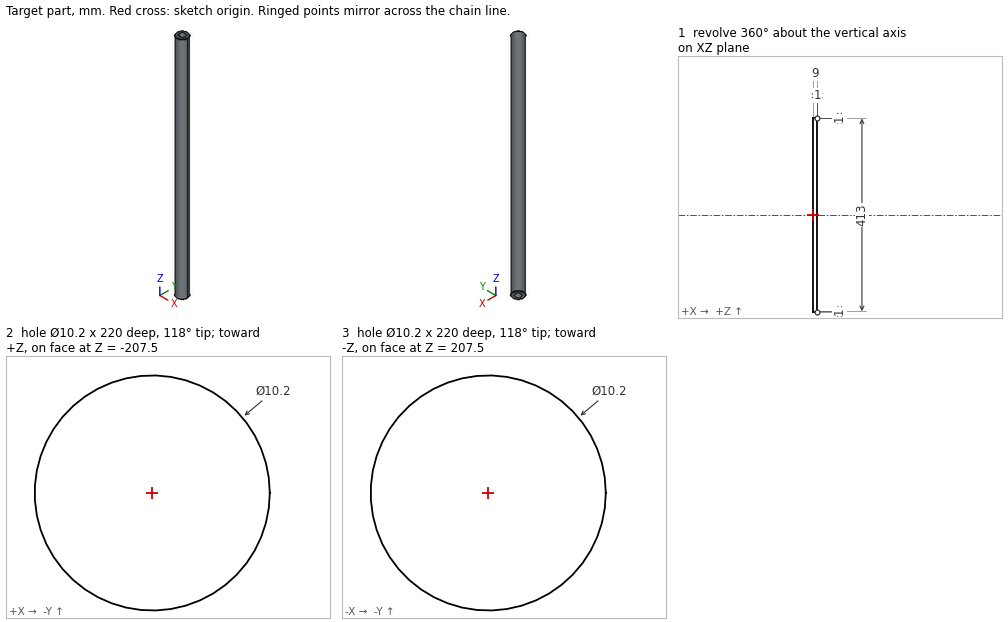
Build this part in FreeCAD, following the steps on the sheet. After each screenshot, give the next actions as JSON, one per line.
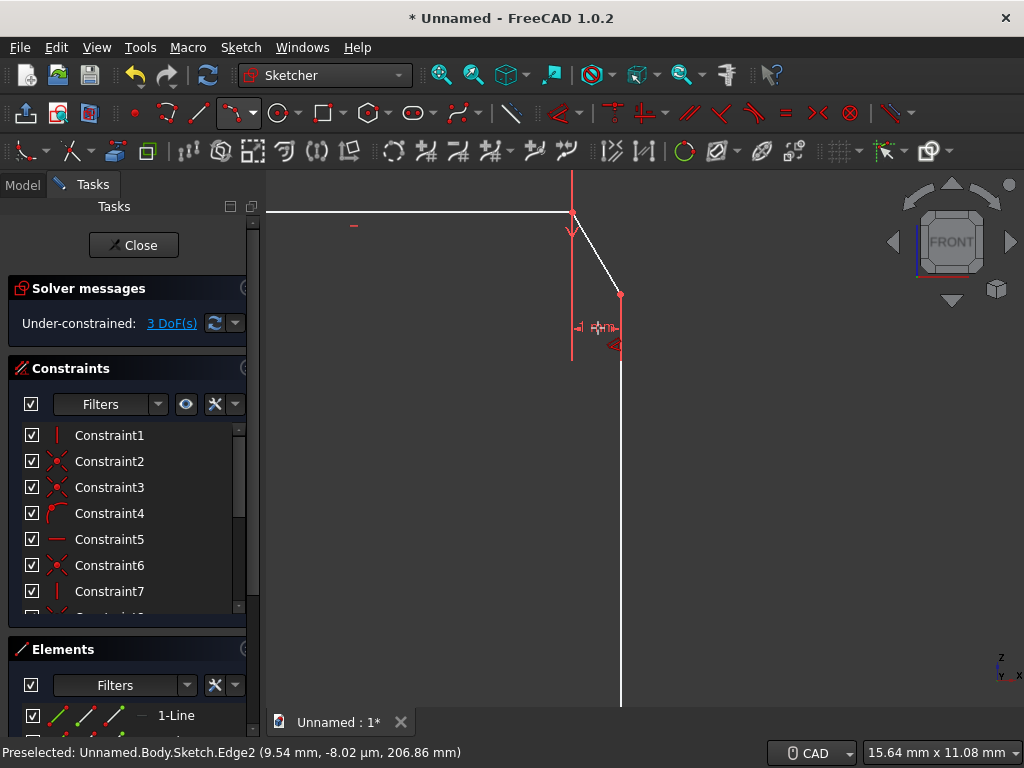
{"action": "left_click", "coordinate": [606, 270]}
{"action": "left_click", "coordinate": [655, 253]}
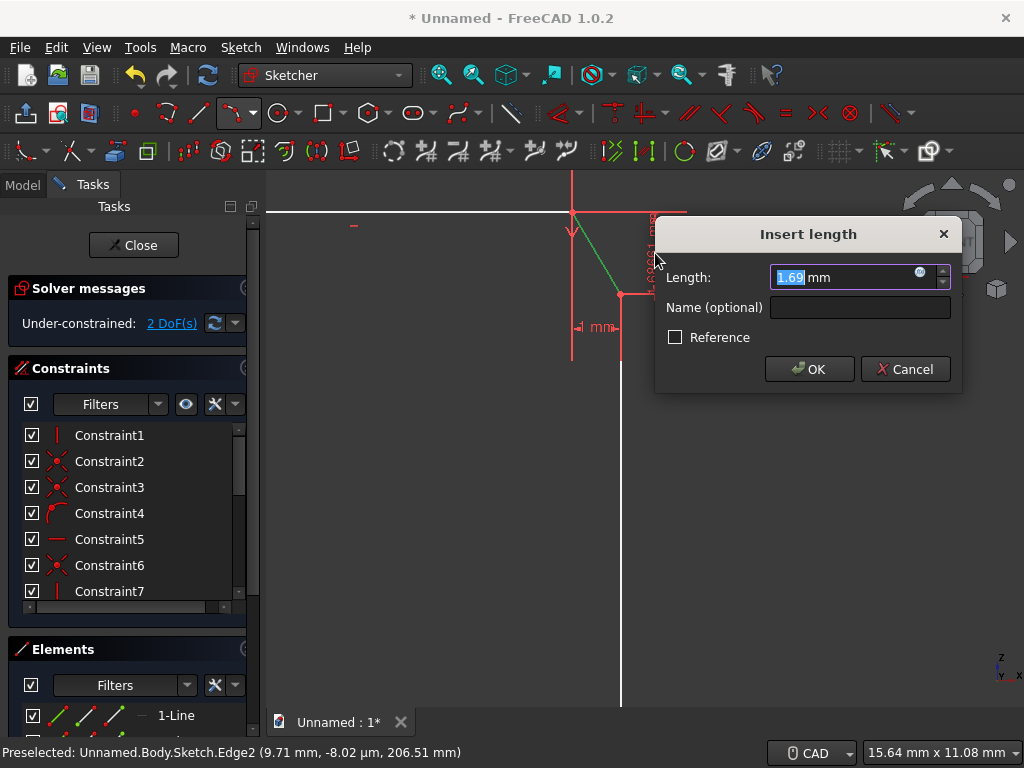
{"action": "type", "text": "1"}
{"action": "key", "text": "Return"}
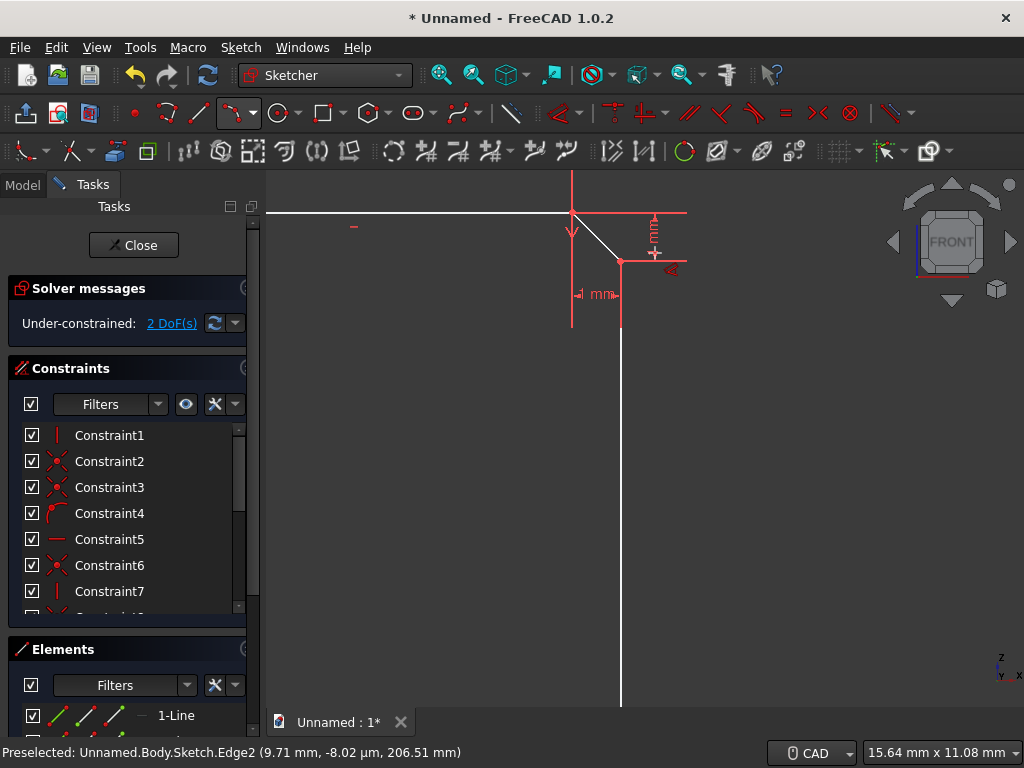
{"action": "scroll", "coordinate": [576, 438], "scroll_direction": "down", "scroll_amount": 15}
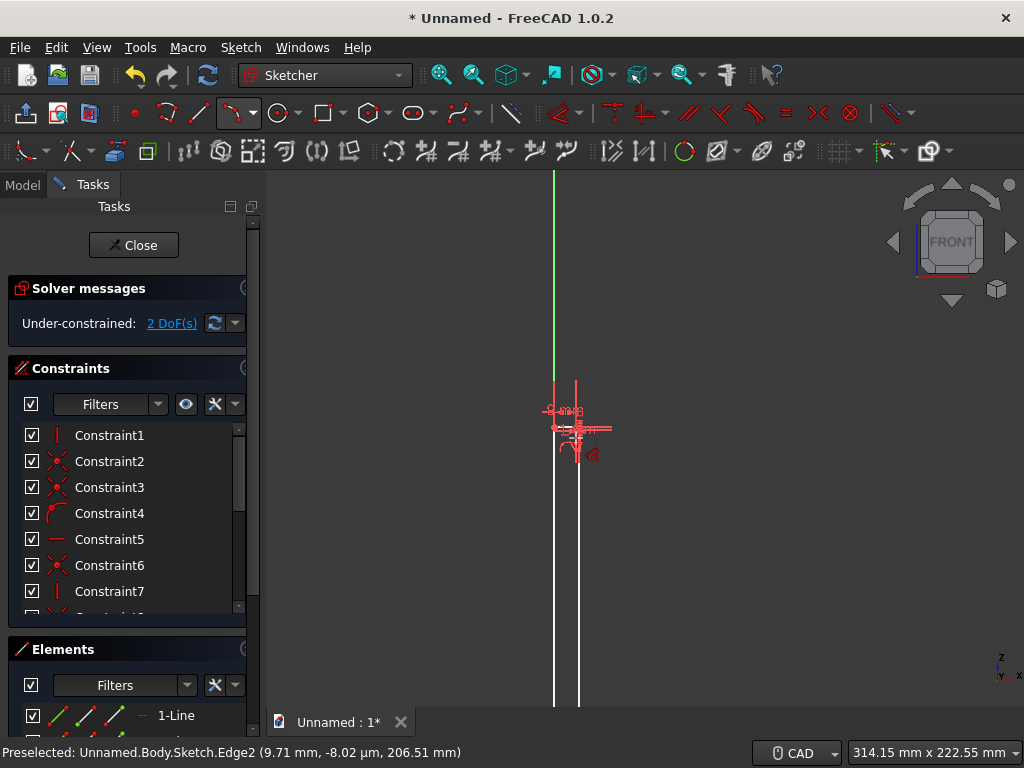
{"action": "scroll", "coordinate": [582, 198], "scroll_direction": "down", "scroll_amount": 5}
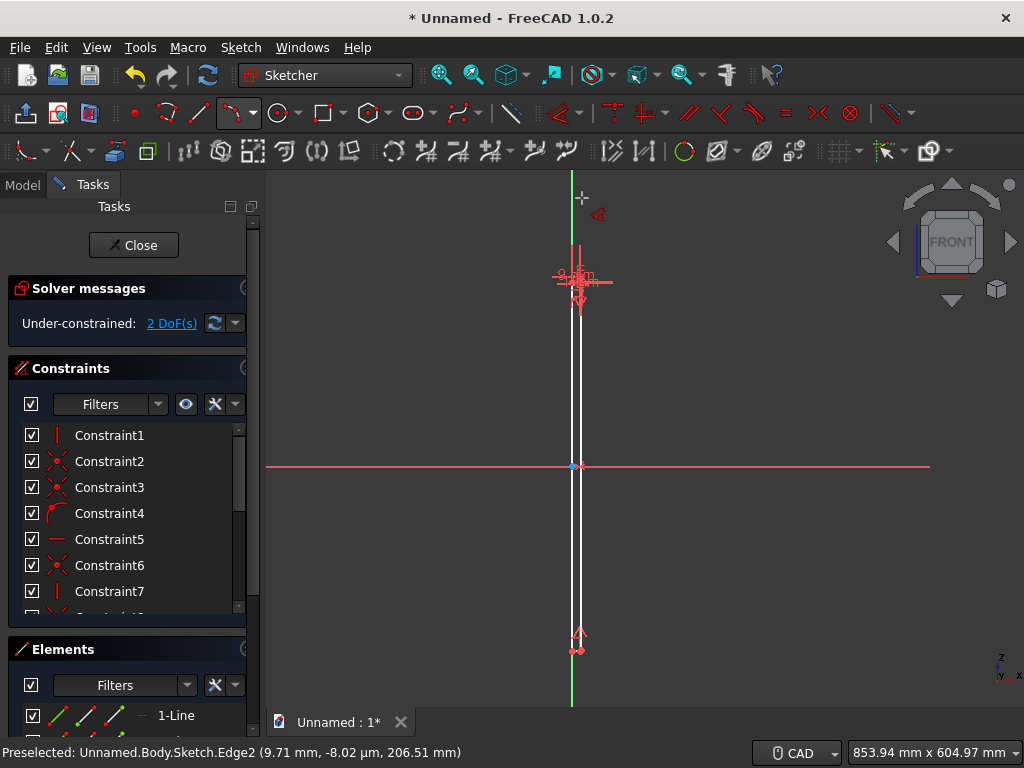
{"action": "scroll", "coordinate": [580, 651], "scroll_direction": "up", "scroll_amount": 20}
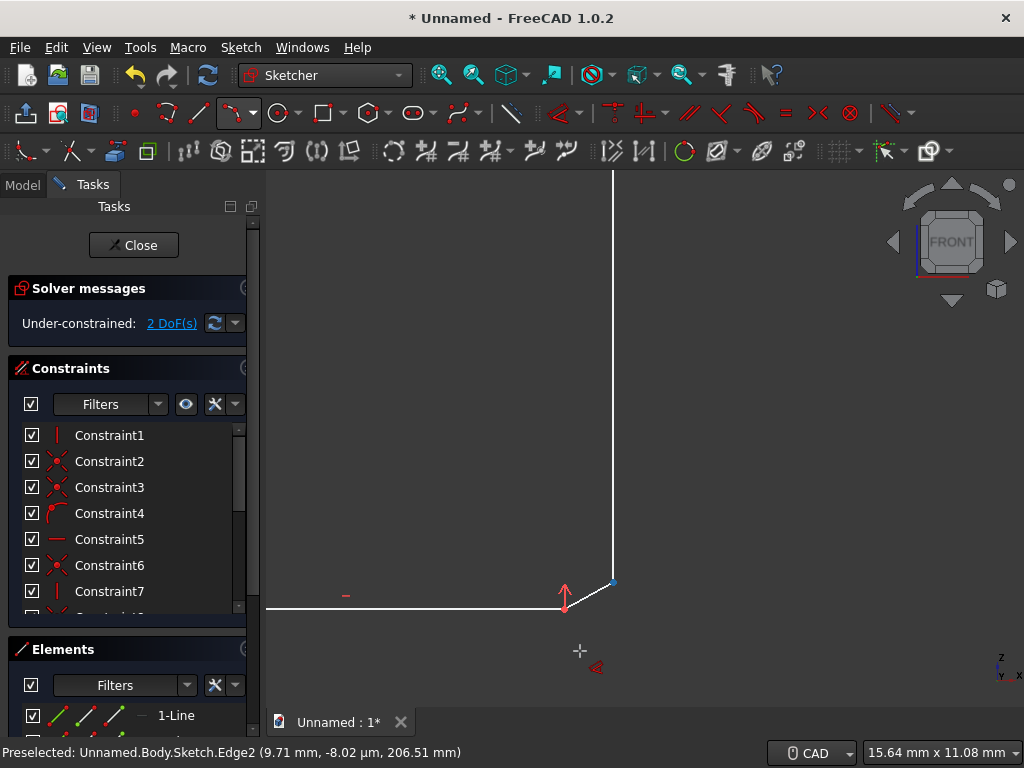
{"action": "left_click", "coordinate": [579, 601]}
{"action": "left_click", "coordinate": [647, 596]}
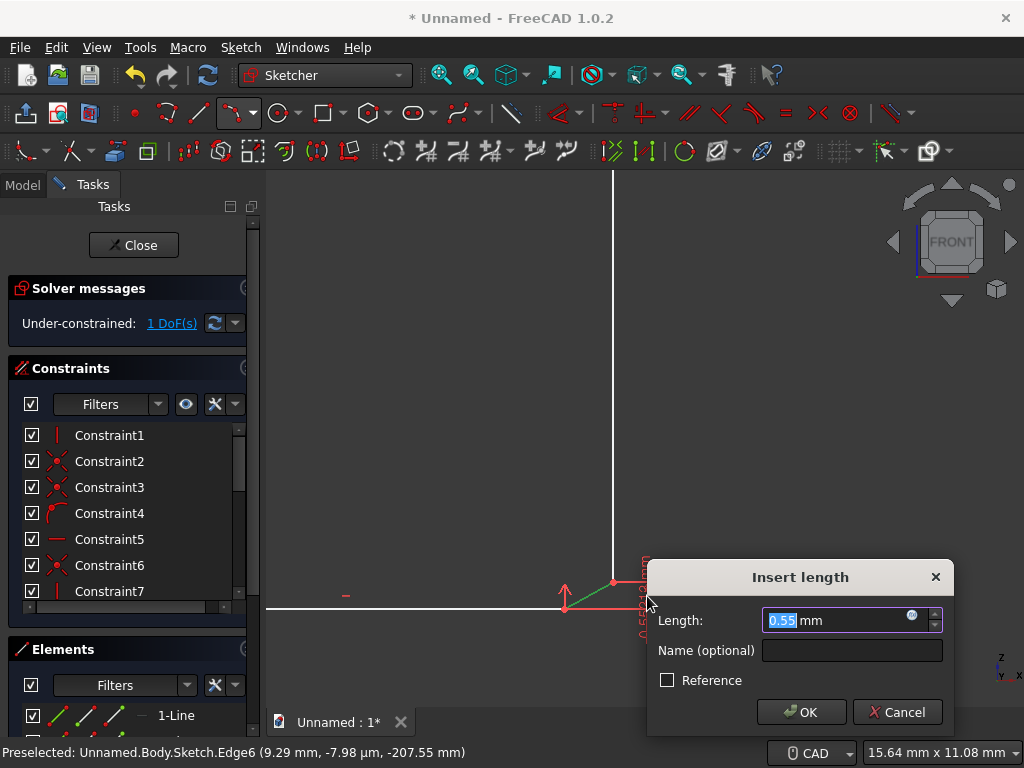
{"action": "type", "text": "1"}
{"action": "key", "text": "Return"}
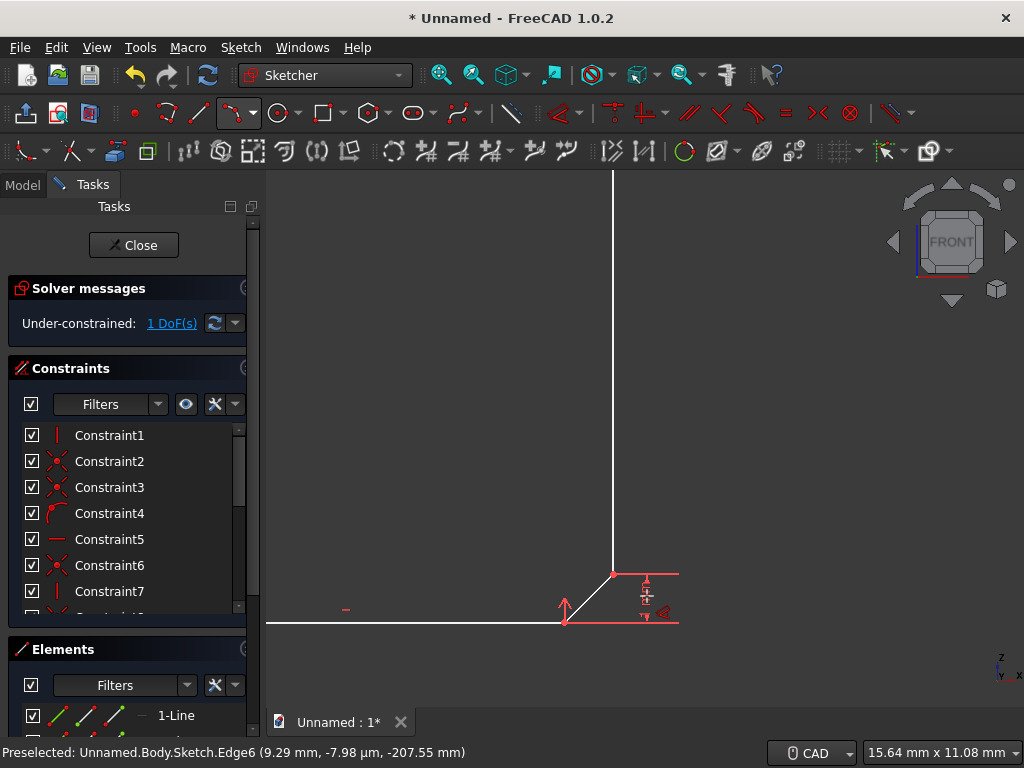
{"action": "scroll", "coordinate": [576, 438], "scroll_direction": "down", "scroll_amount": 15}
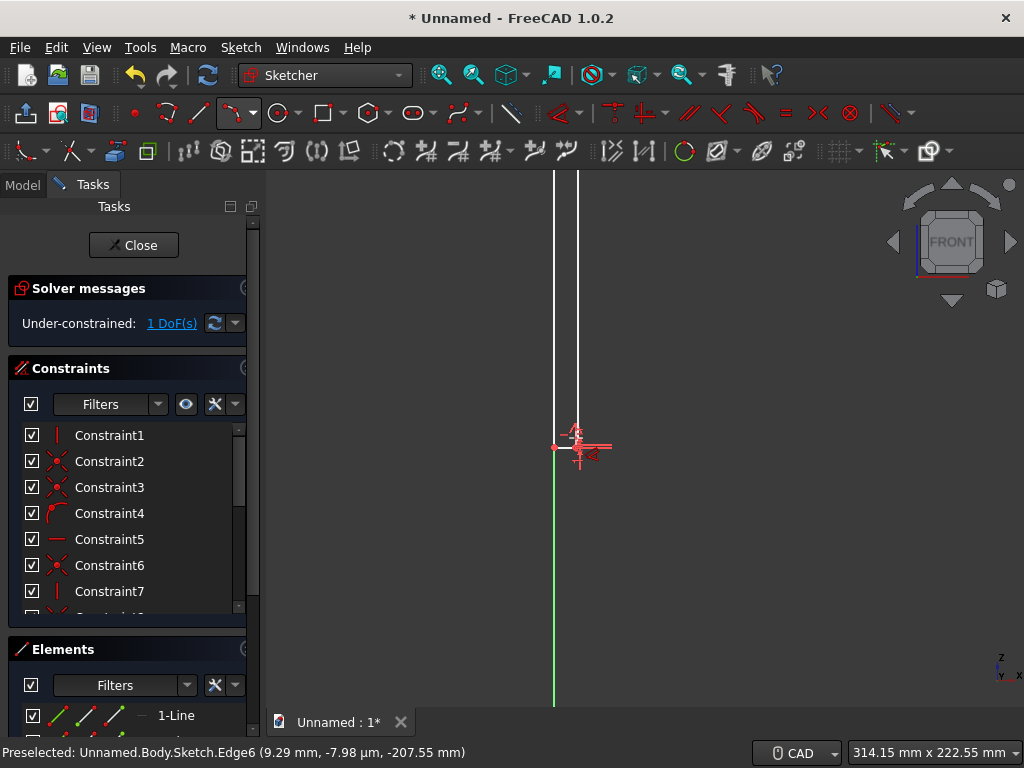
{"action": "scroll", "coordinate": [583, 679], "scroll_direction": "down", "scroll_amount": 5}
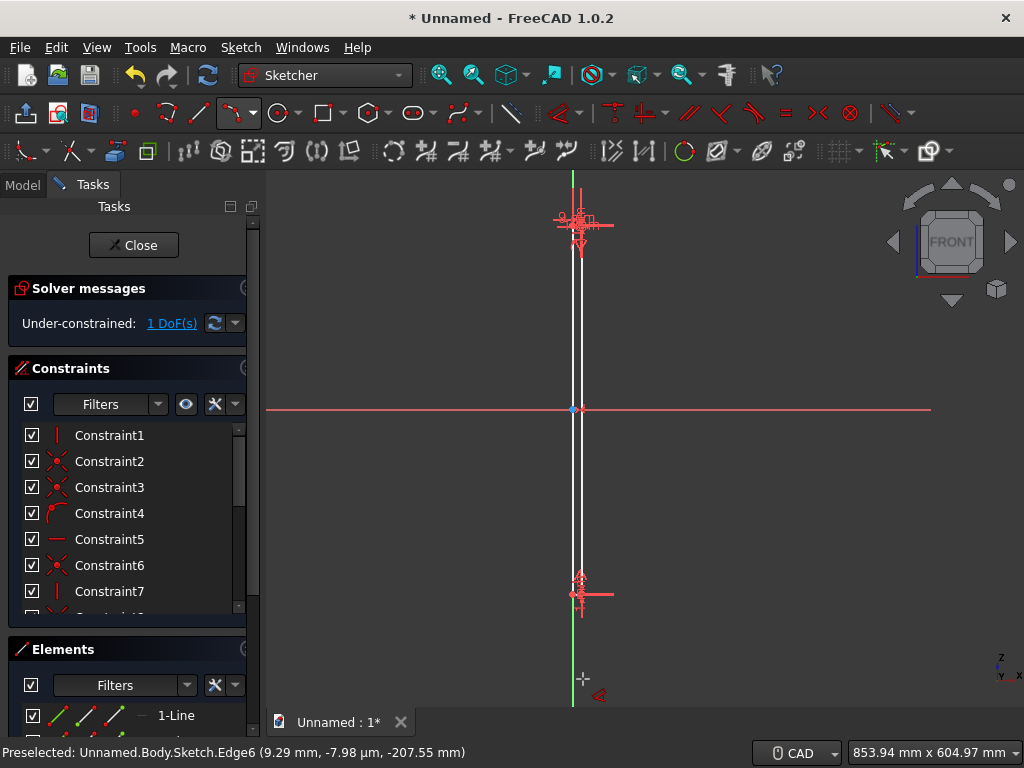
{"action": "scroll", "coordinate": [582, 483], "scroll_direction": "up", "scroll_amount": 3}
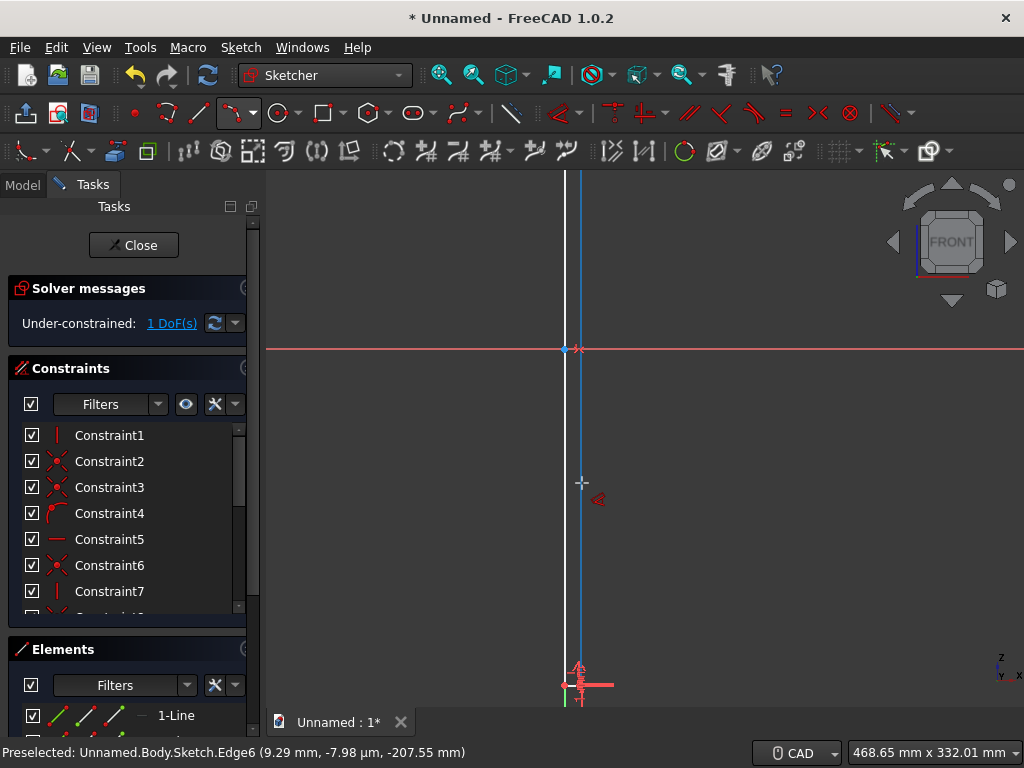
{"action": "left_click", "coordinate": [581, 483]}
{"action": "left_click", "coordinate": [615, 438]}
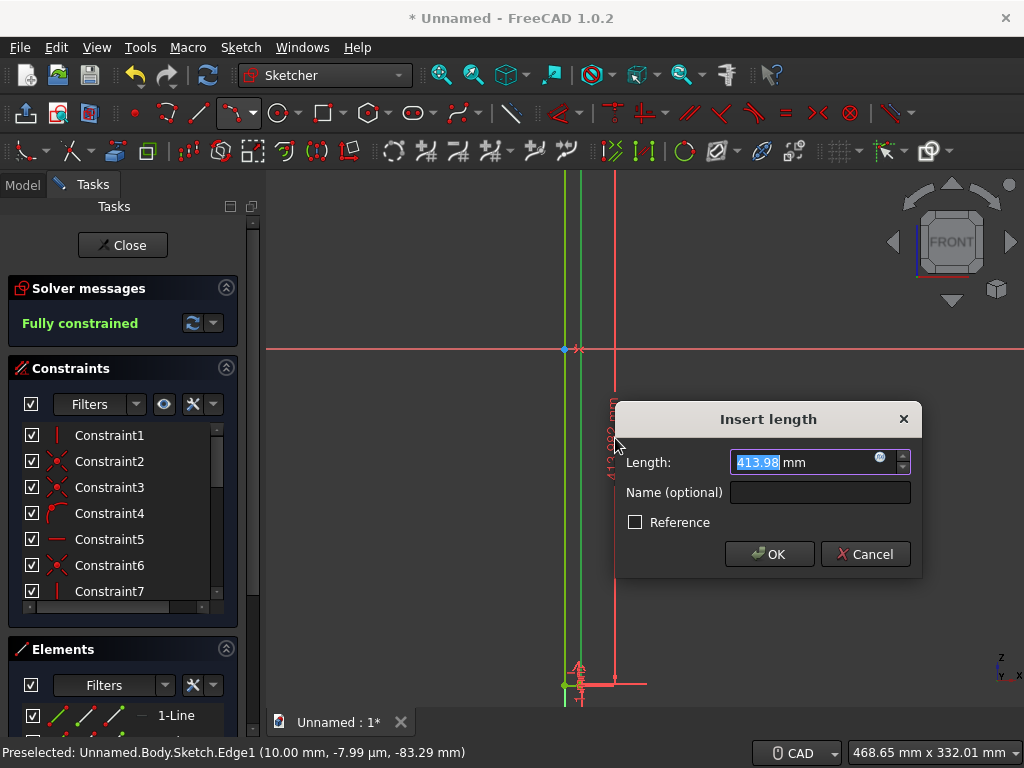
{"action": "type", "text": "413"}
{"action": "key", "text": "Return"}
{"action": "key", "text": "Escape"}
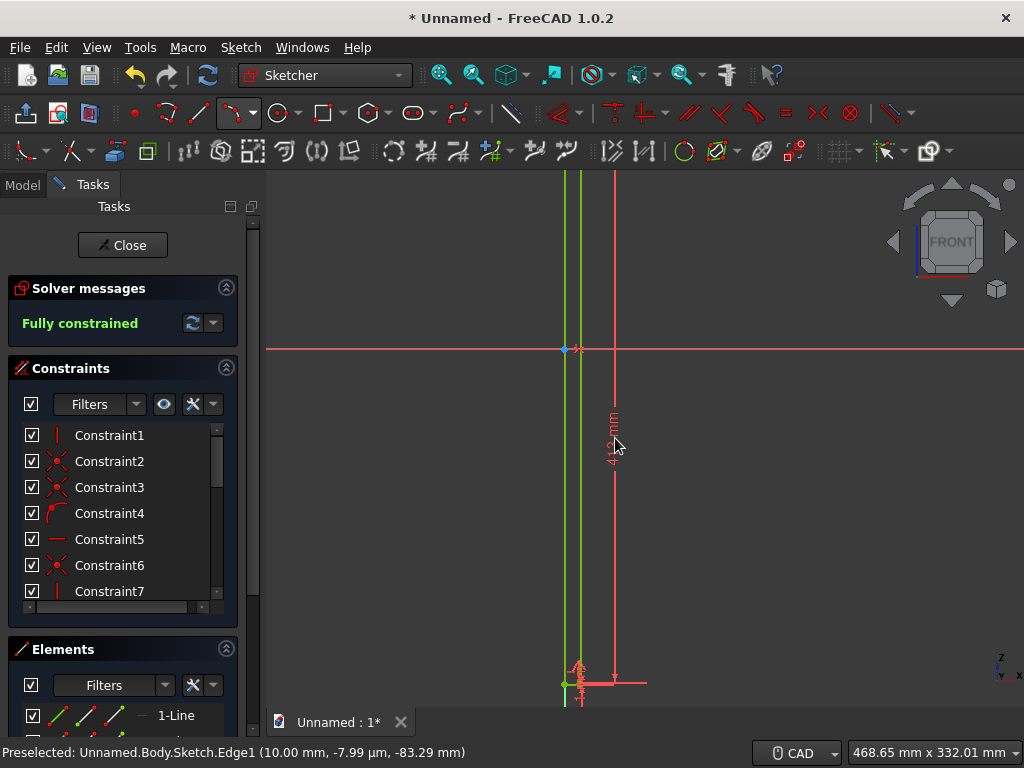
{"action": "left_click", "coordinate": [123, 245]}